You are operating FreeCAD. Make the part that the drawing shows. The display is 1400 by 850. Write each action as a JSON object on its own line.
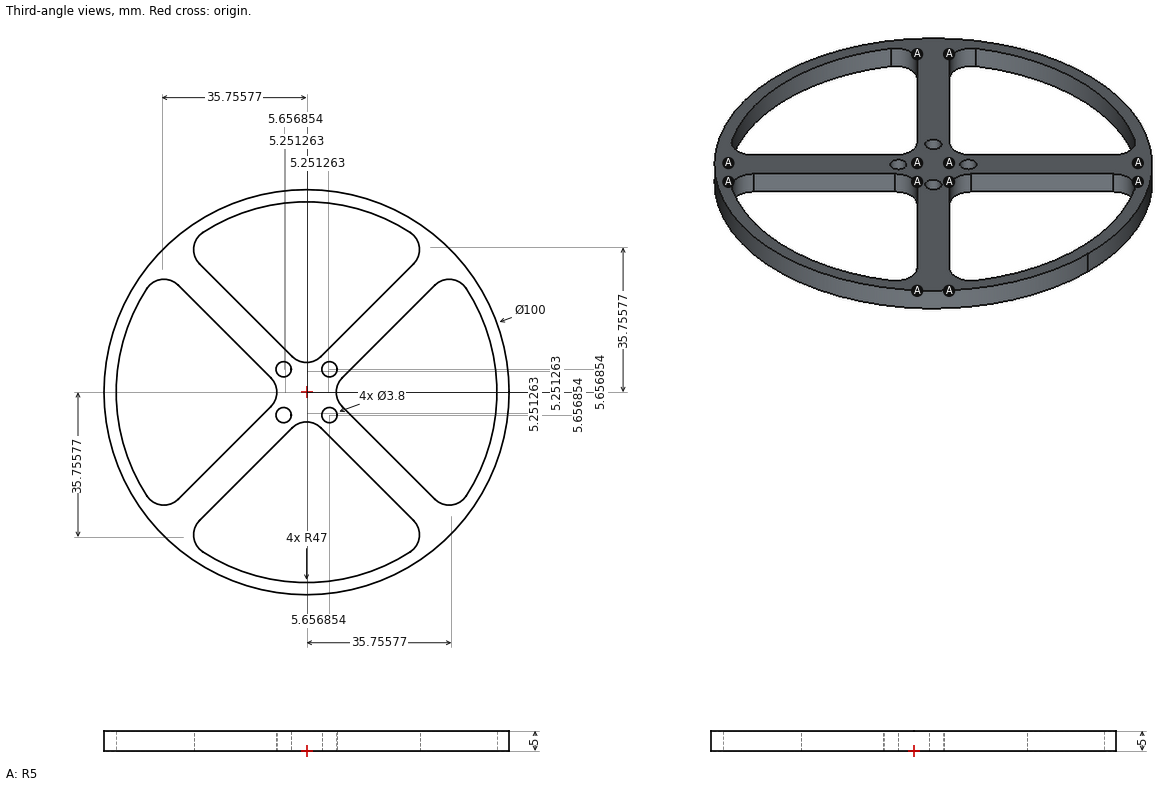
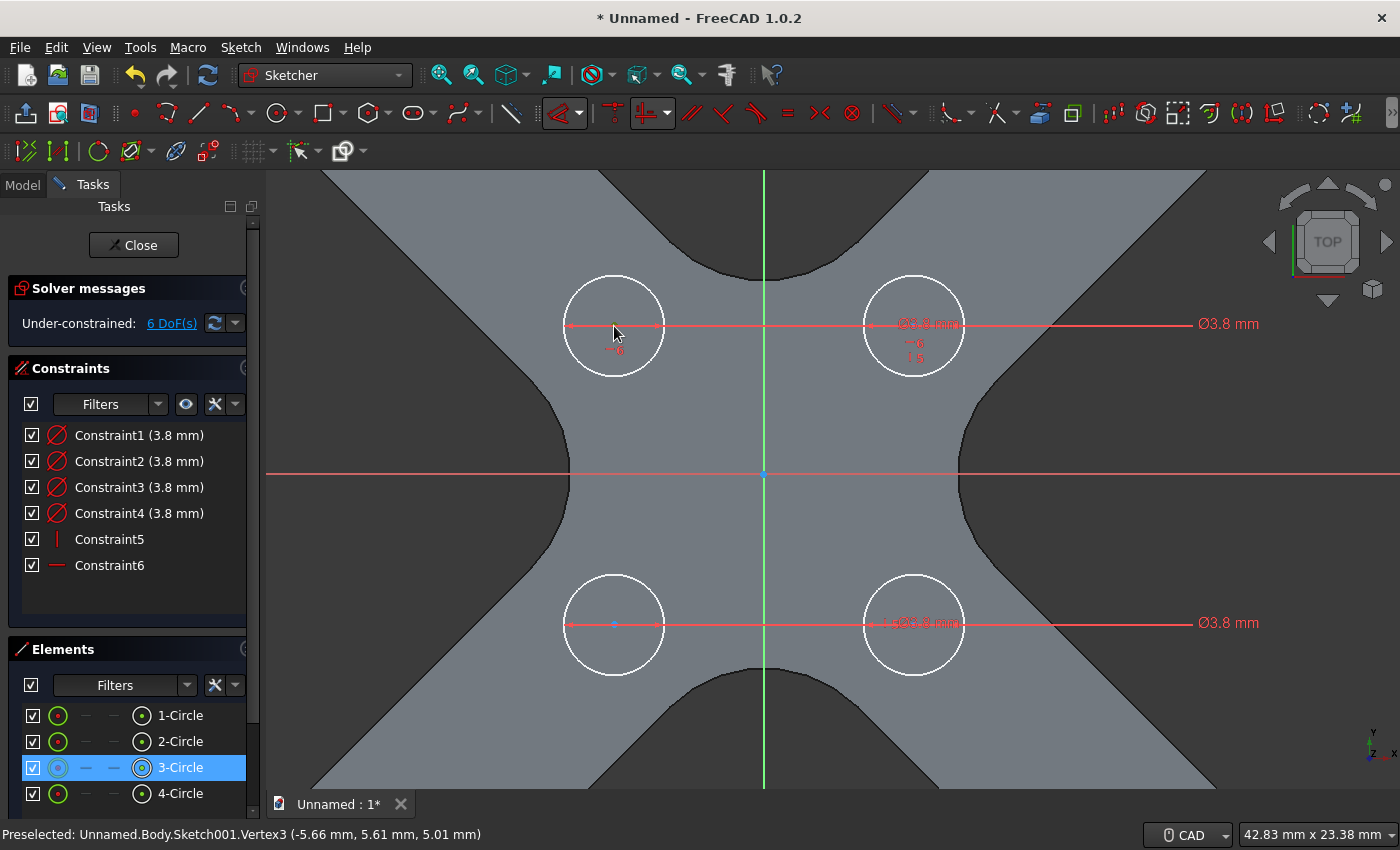
{"action": "left_click", "coordinate": [614, 625]}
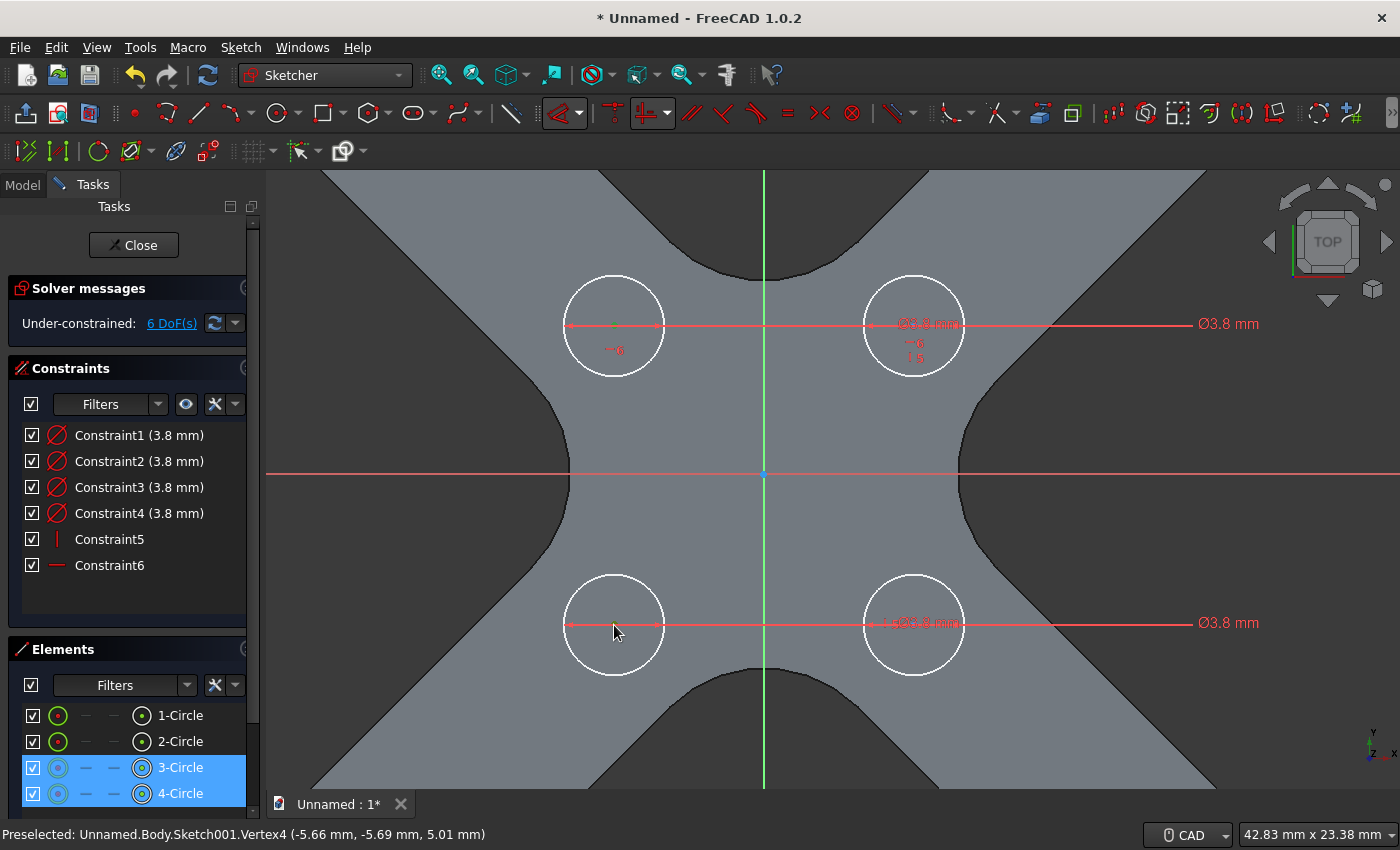
{"action": "left_click", "coordinate": [670, 114]}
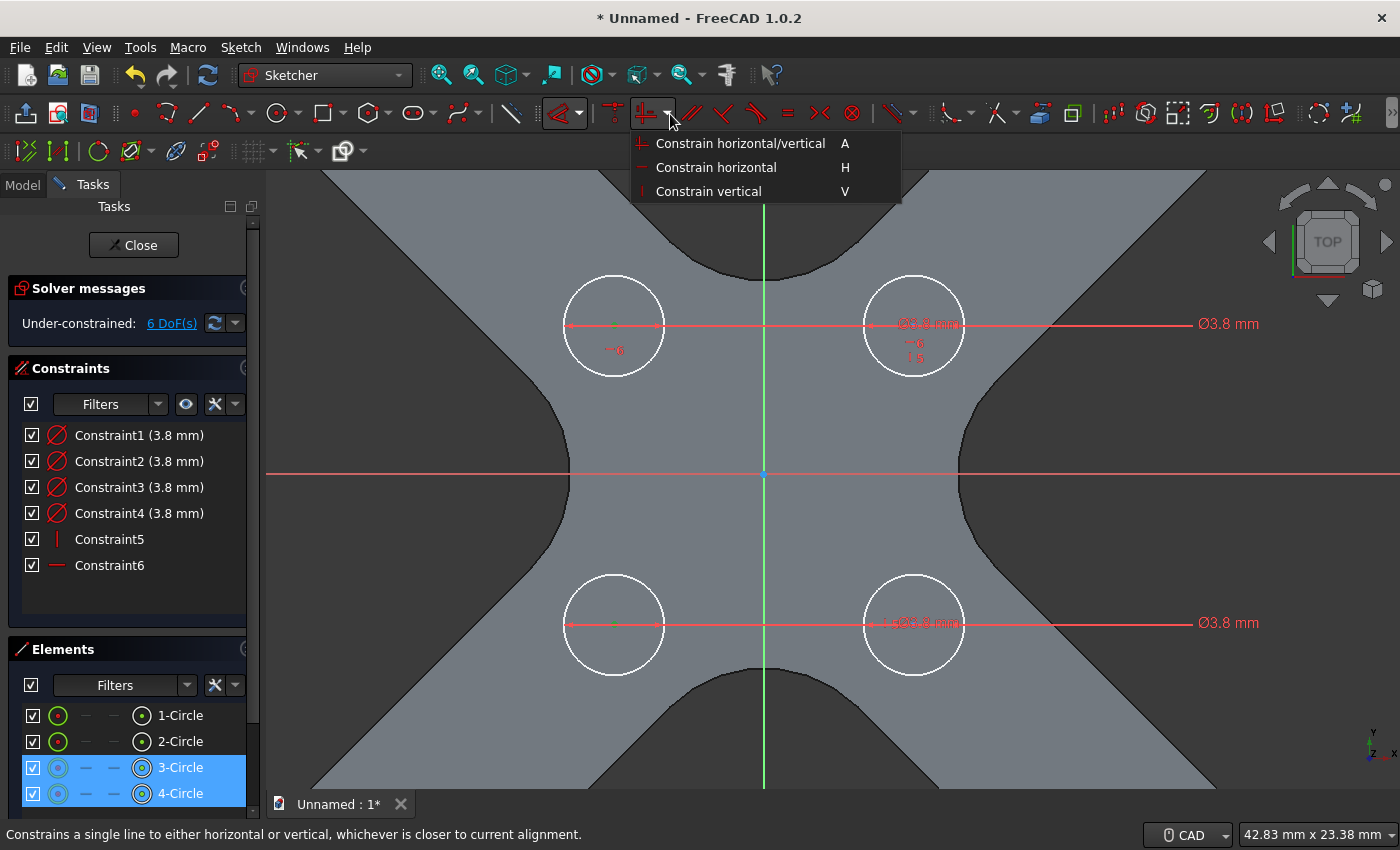
{"action": "left_click", "coordinate": [766, 191]}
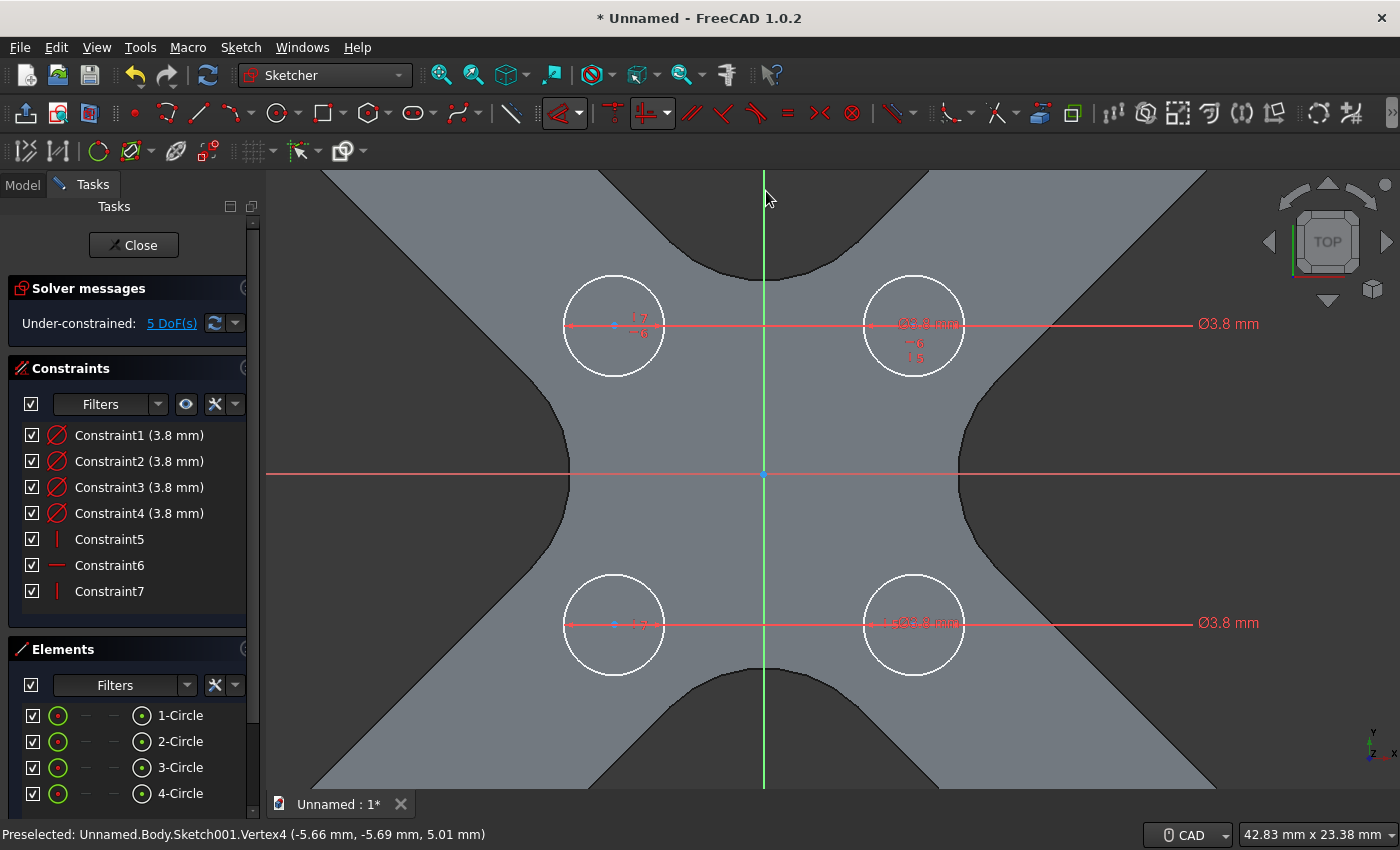
{"action": "left_click", "coordinate": [914, 625]}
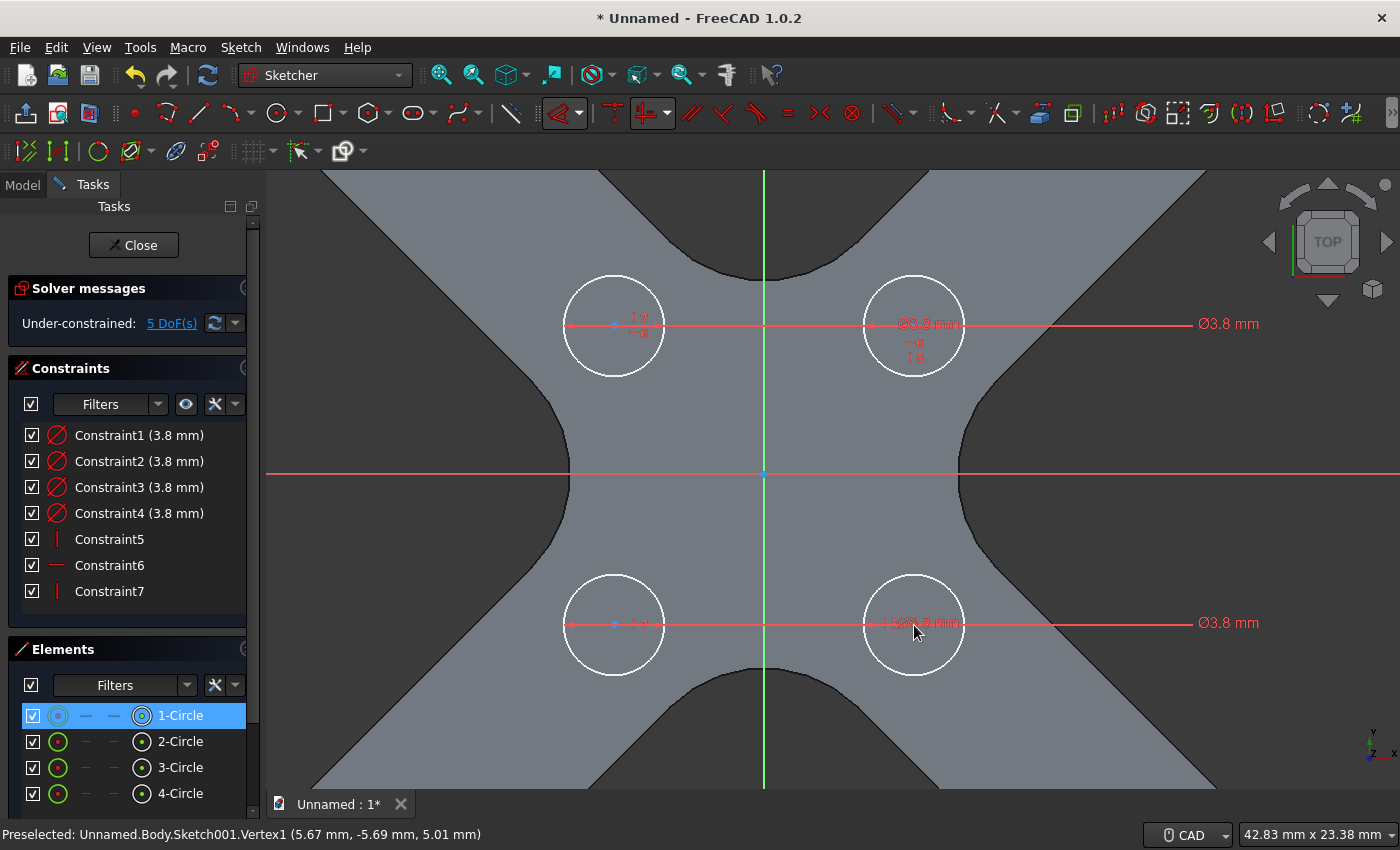
{"action": "left_click", "coordinate": [614, 625]}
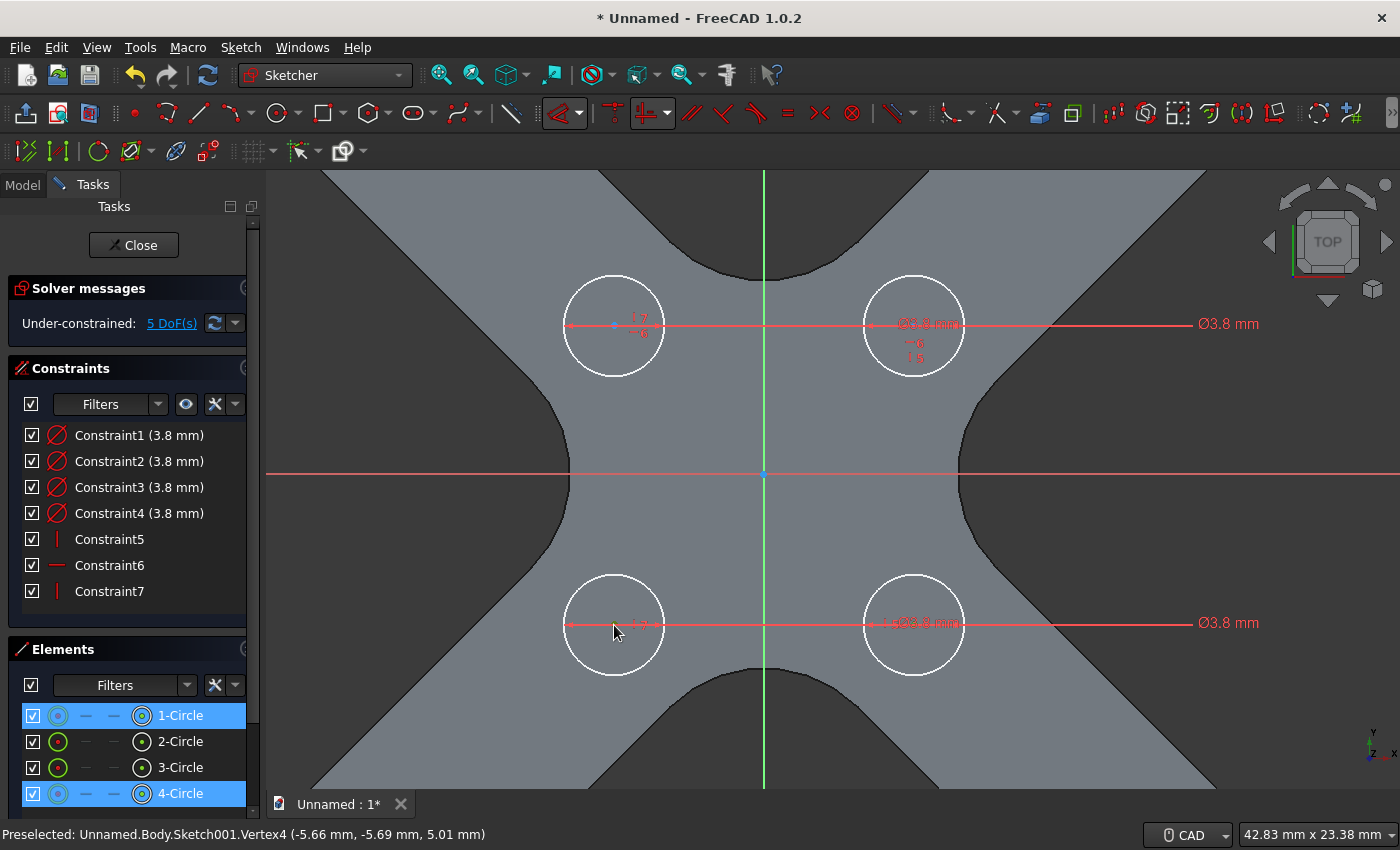
{"action": "left_click", "coordinate": [670, 114]}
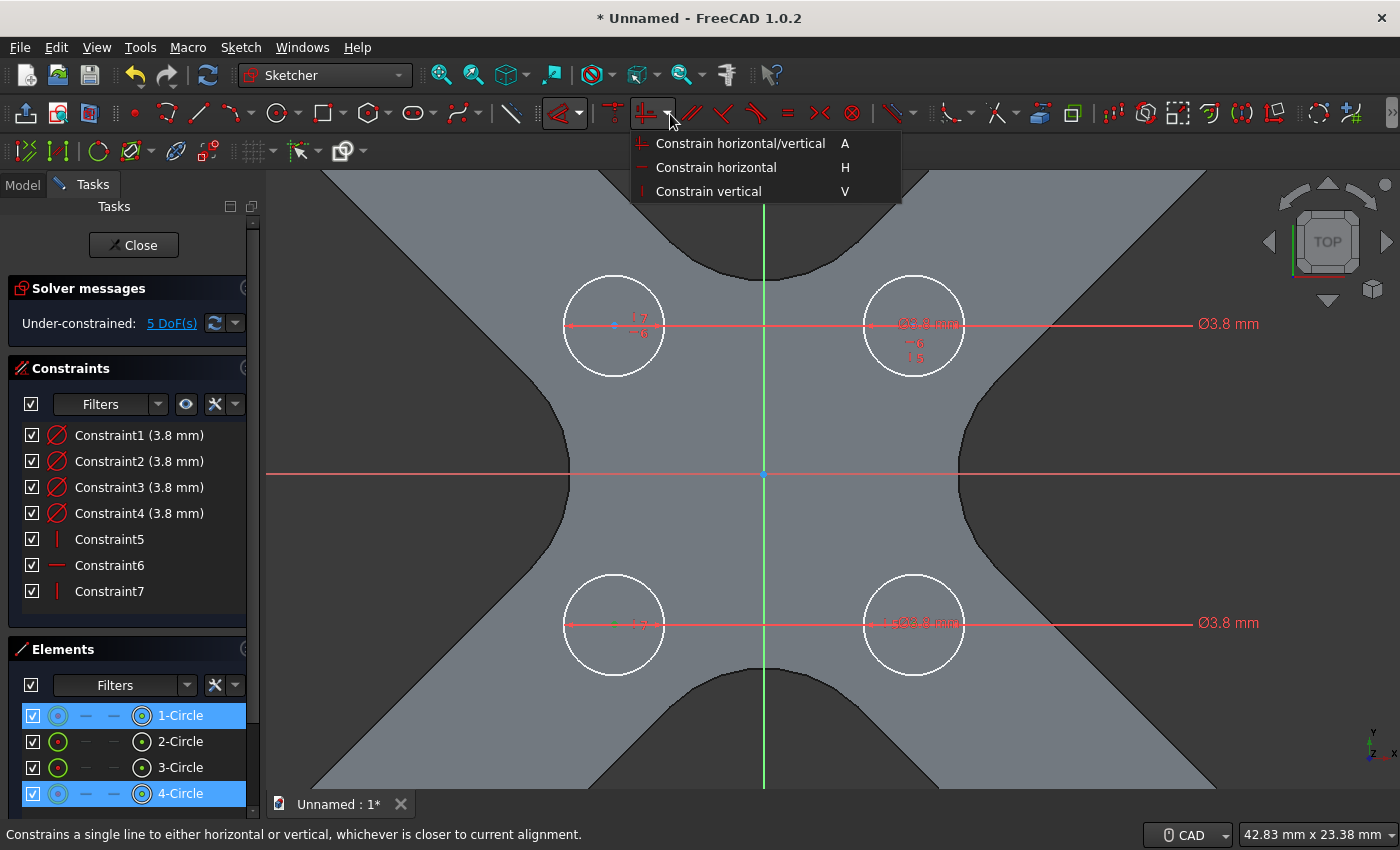
{"action": "left_click", "coordinate": [766, 167]}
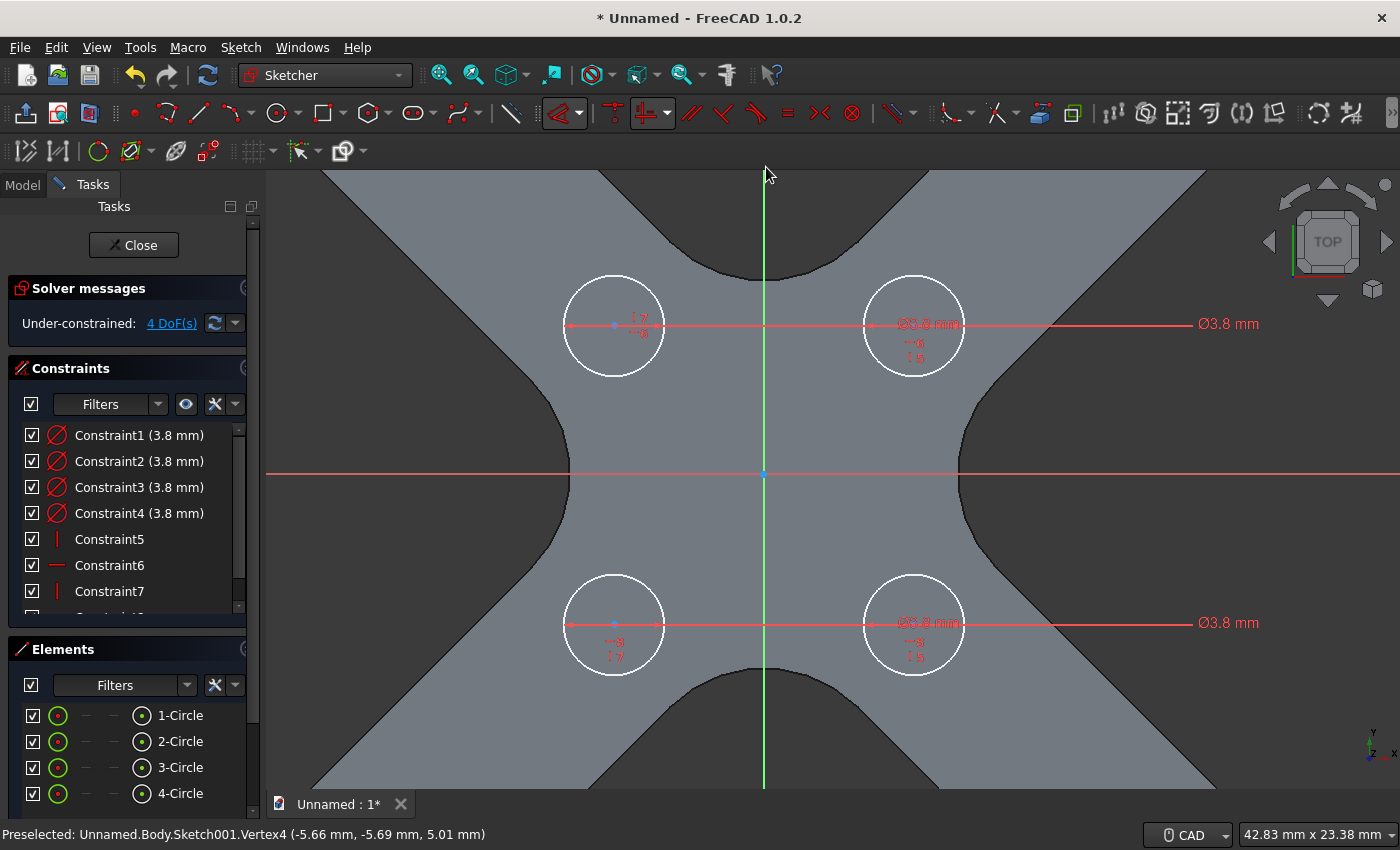
{"action": "left_click", "coordinate": [914, 625]}